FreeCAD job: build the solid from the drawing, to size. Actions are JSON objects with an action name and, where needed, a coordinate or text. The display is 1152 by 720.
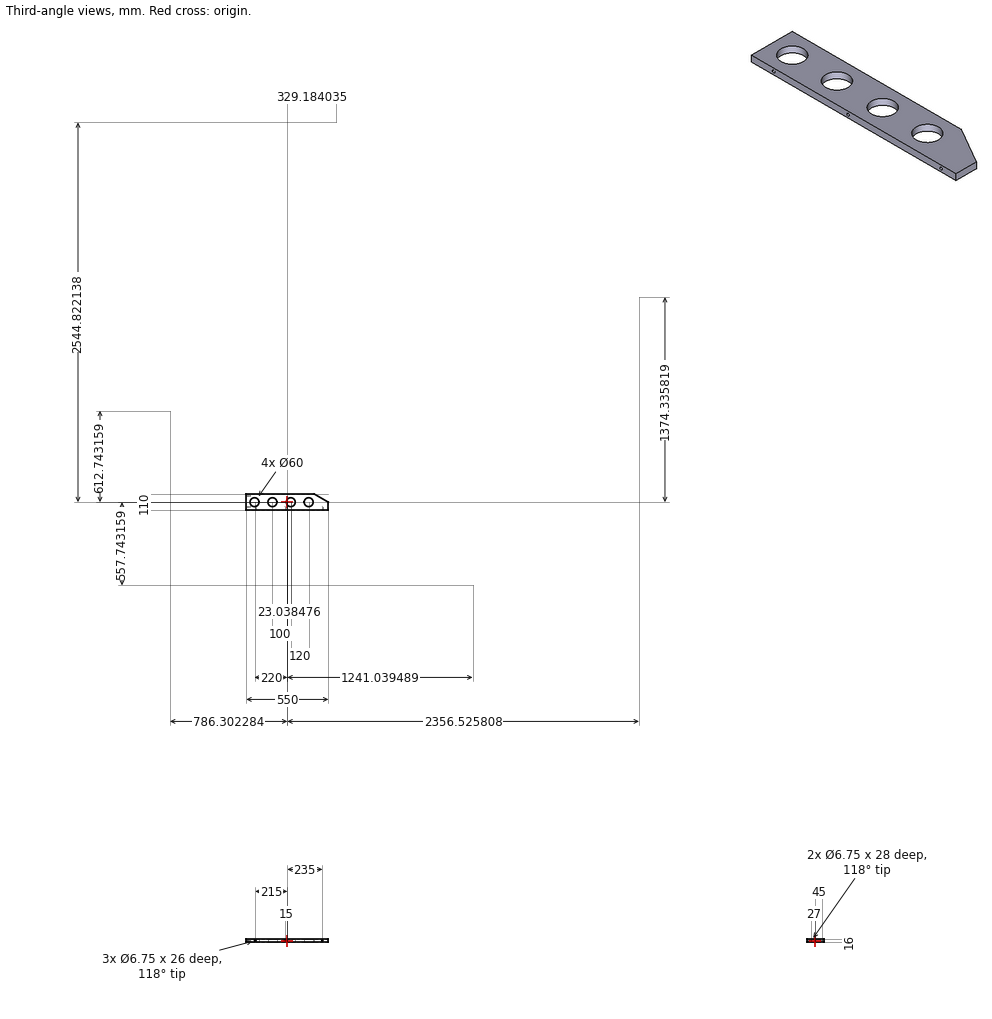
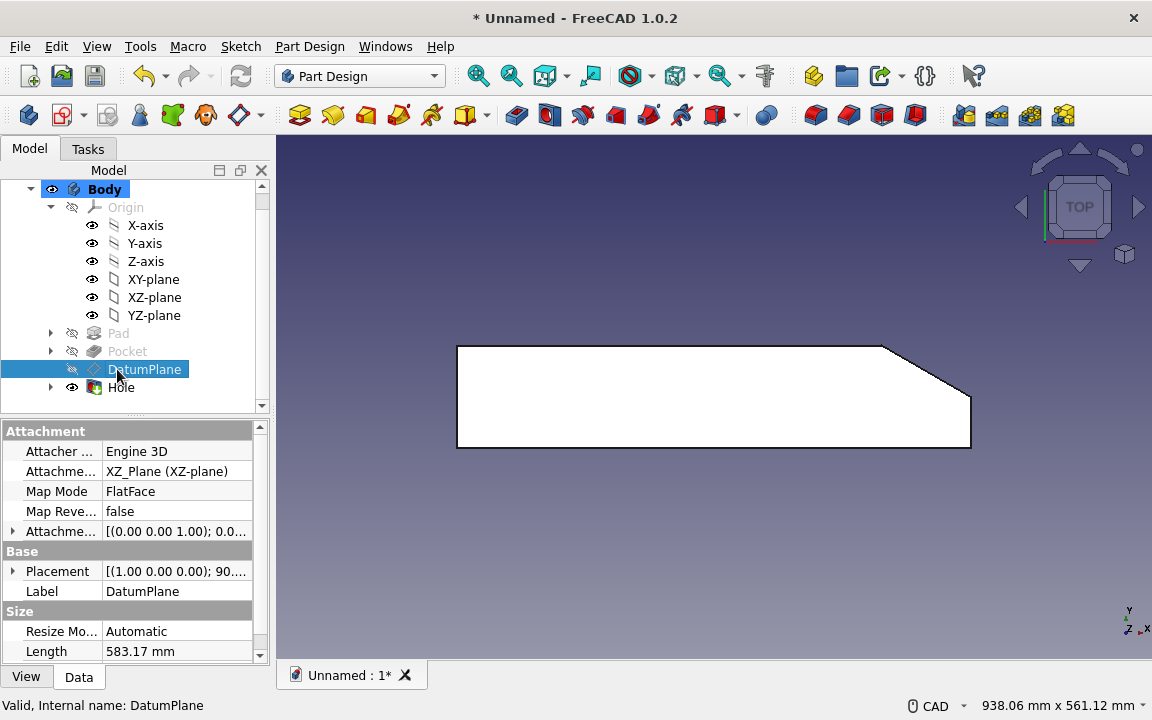
{"action": "key", "text": "6"}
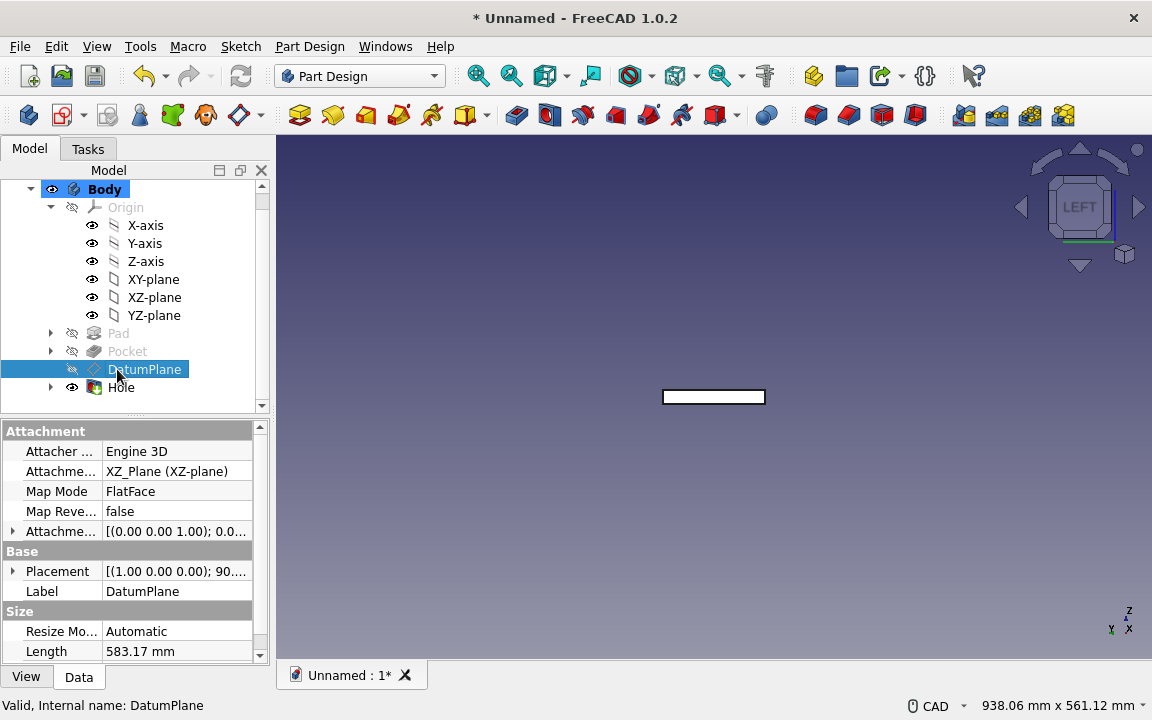
{"action": "key", "text": "v f"}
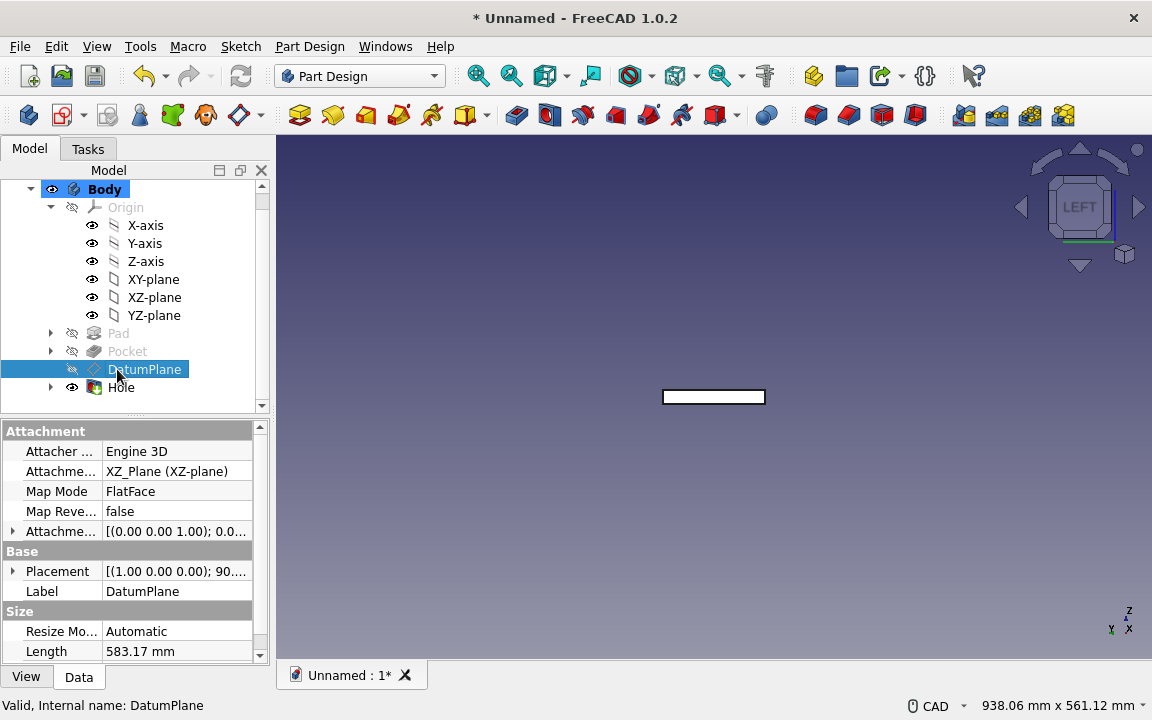
{"action": "key", "text": "2"}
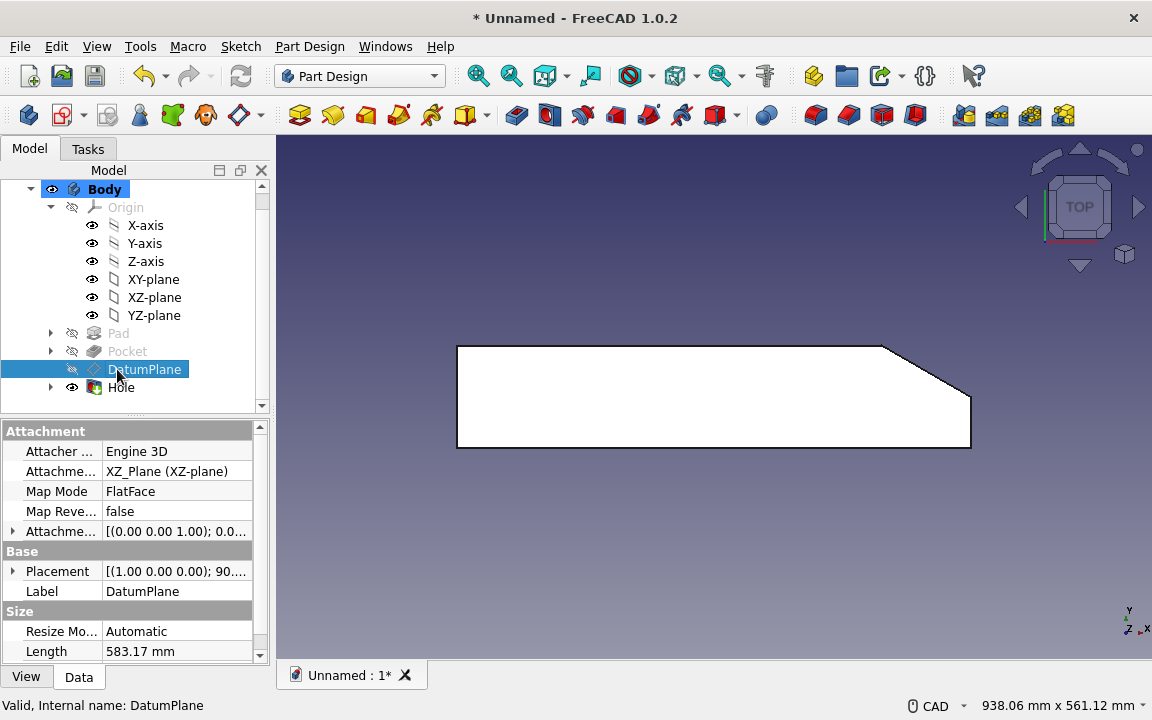
{"action": "key", "text": "1"}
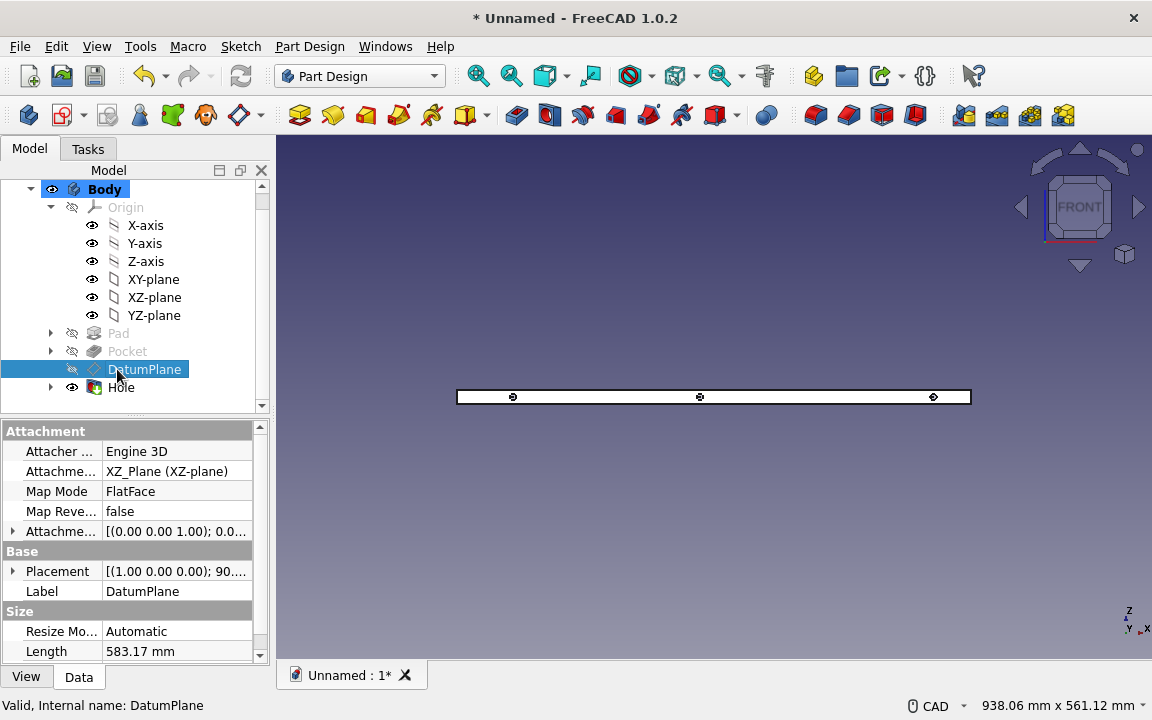
{"action": "left_click", "coordinate": [137, 315]}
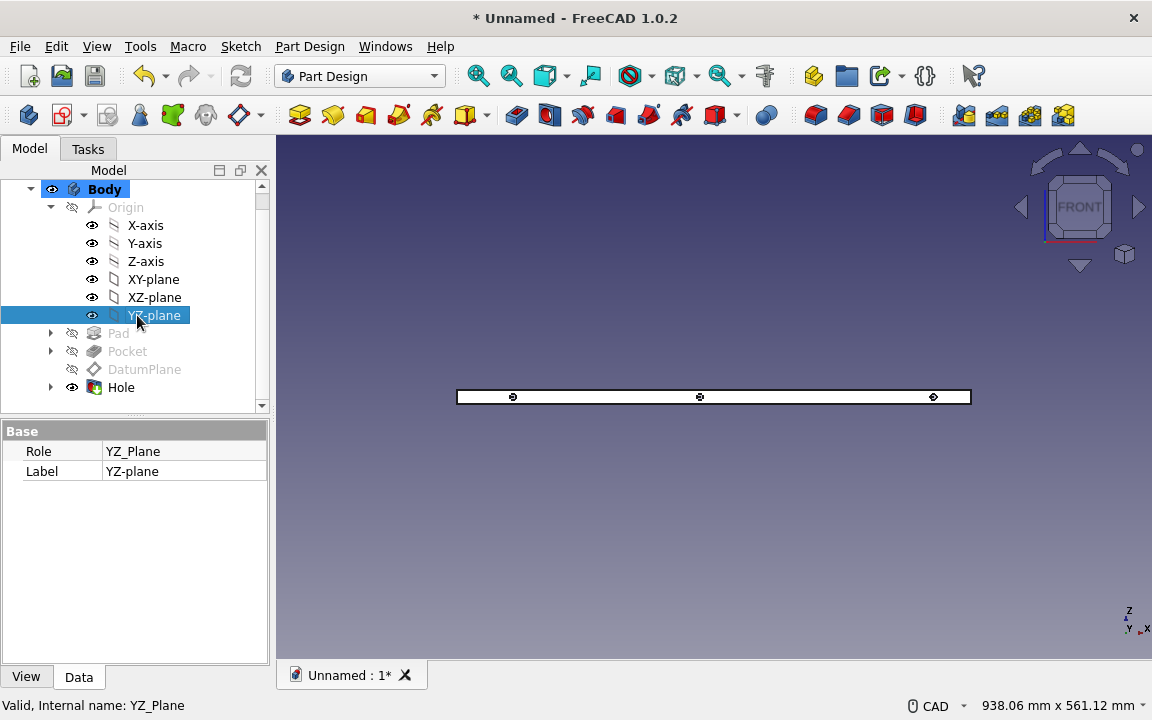
{"action": "left_click", "coordinate": [238, 116]}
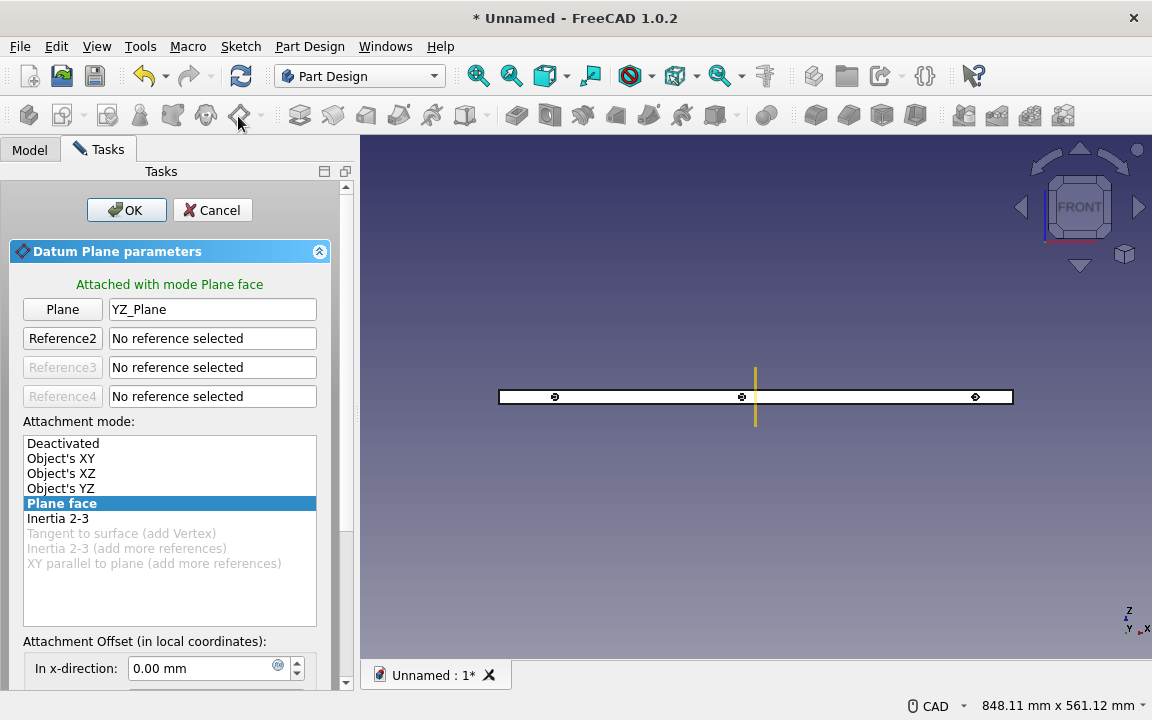
{"action": "scroll", "coordinate": [346, 436], "scroll_direction": "down", "scroll_amount": 2}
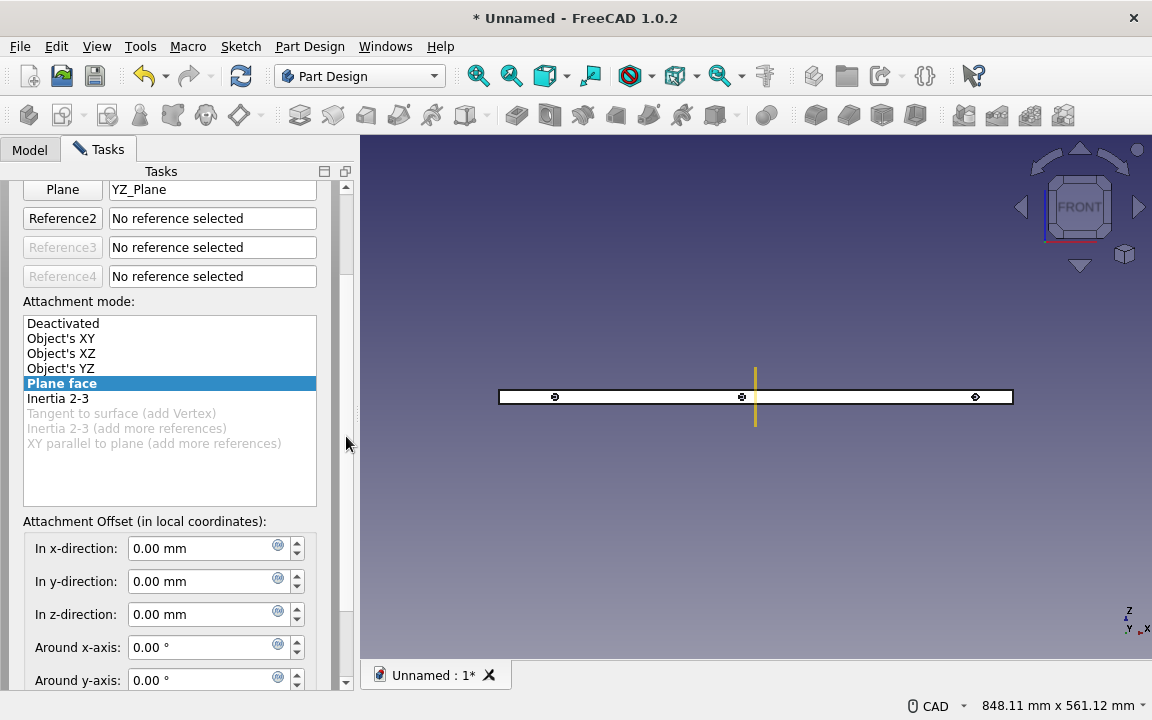
{"action": "triple_click", "coordinate": [210, 614]}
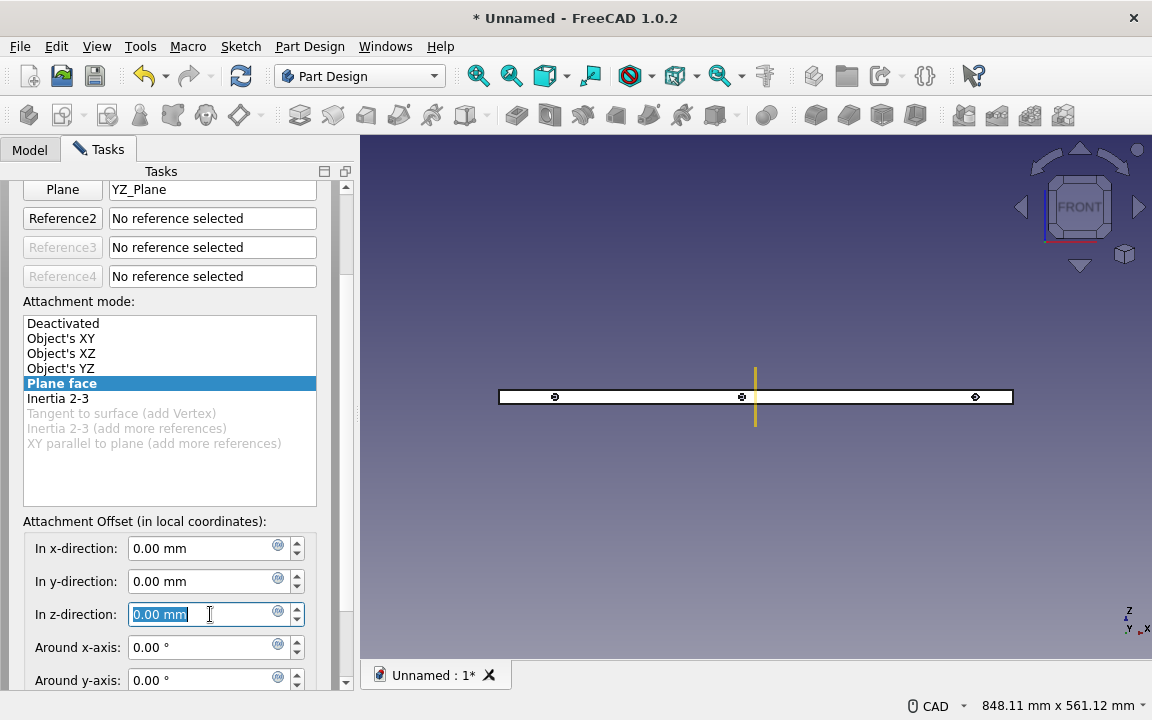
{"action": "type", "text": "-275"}
{"action": "key", "text": "Tab"}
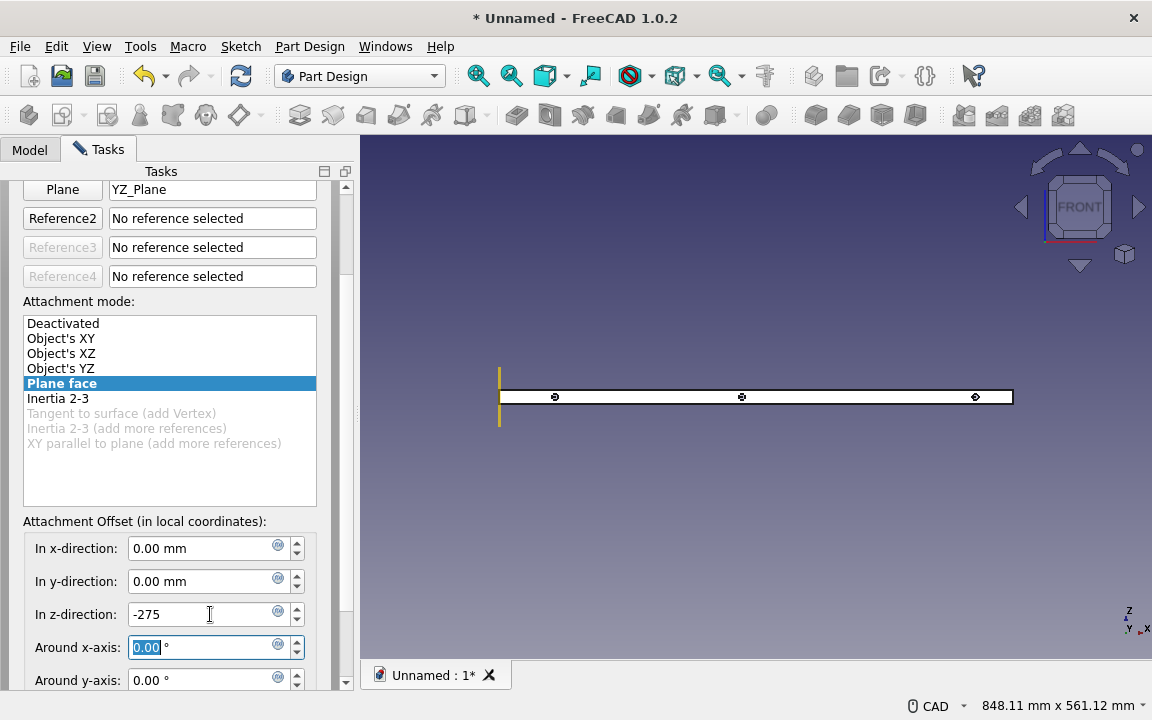
{"action": "scroll", "coordinate": [346, 436], "scroll_direction": "up", "scroll_amount": 3}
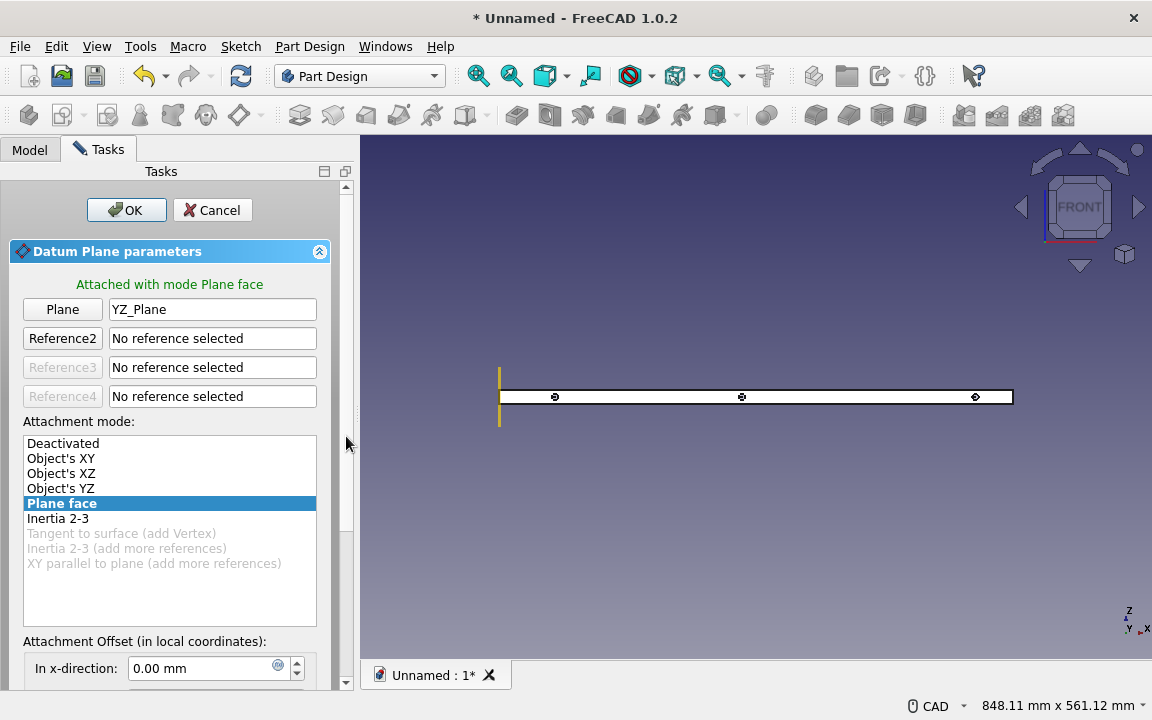
{"action": "left_click", "coordinate": [127, 210]}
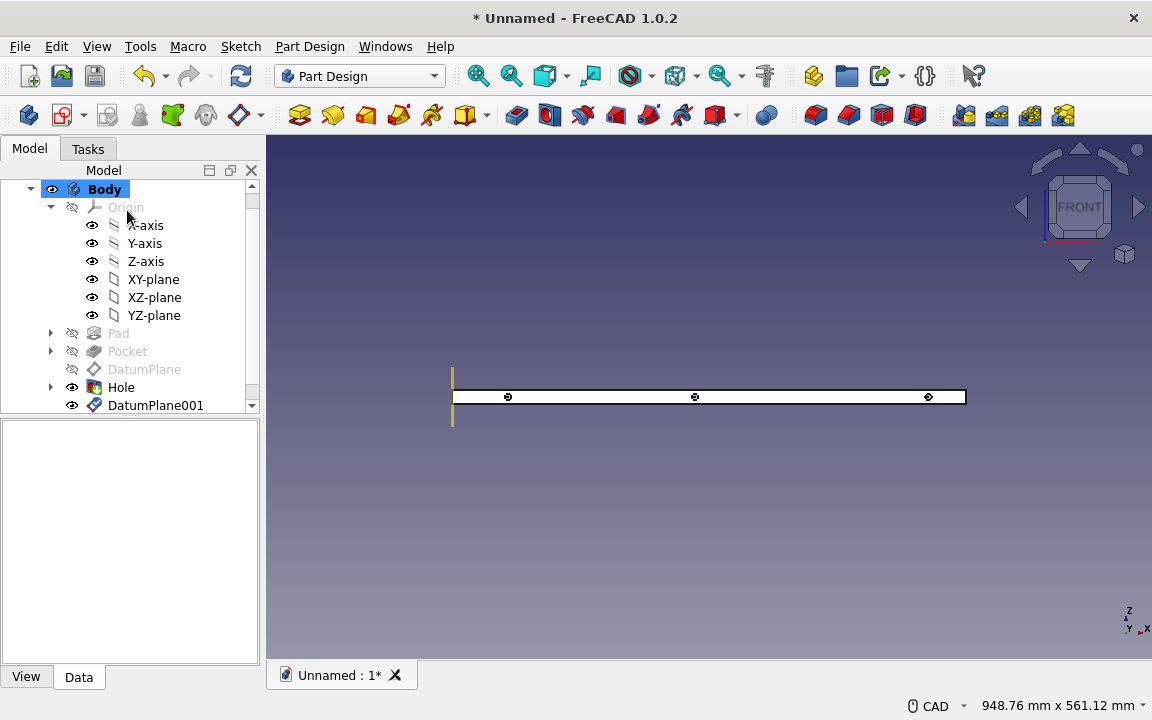
{"action": "left_click", "coordinate": [117, 405]}